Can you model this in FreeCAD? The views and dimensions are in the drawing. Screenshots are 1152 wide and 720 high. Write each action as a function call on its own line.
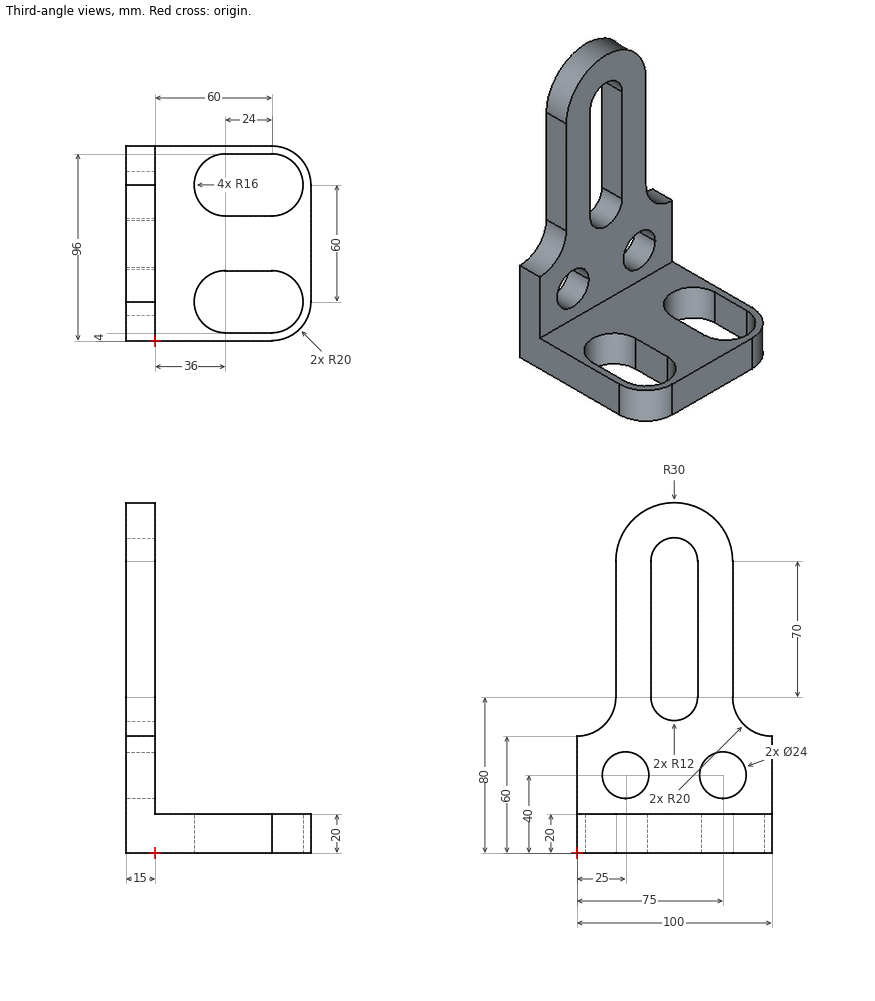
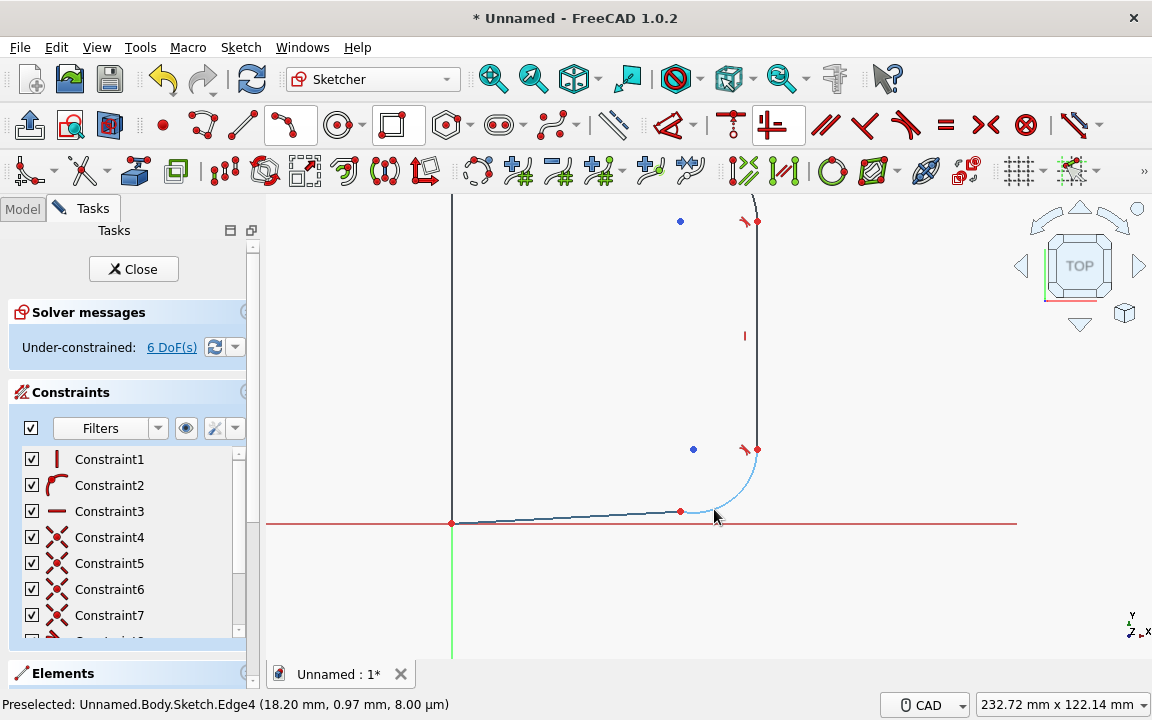
click(714, 509)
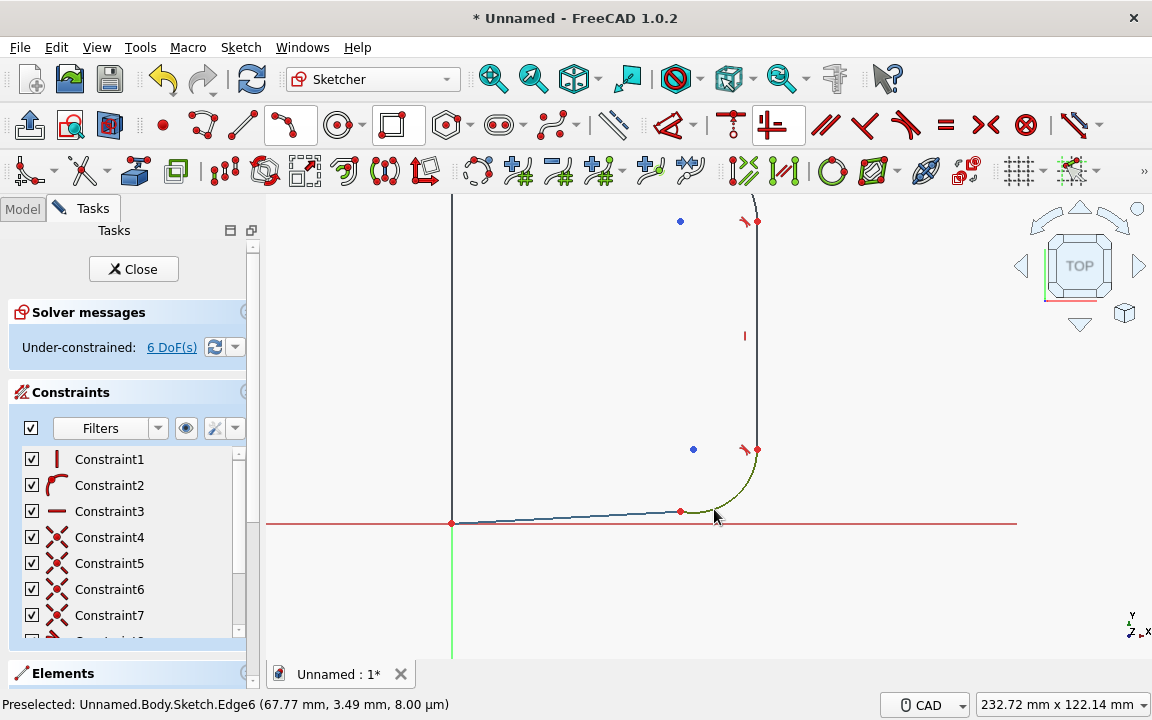
key(t)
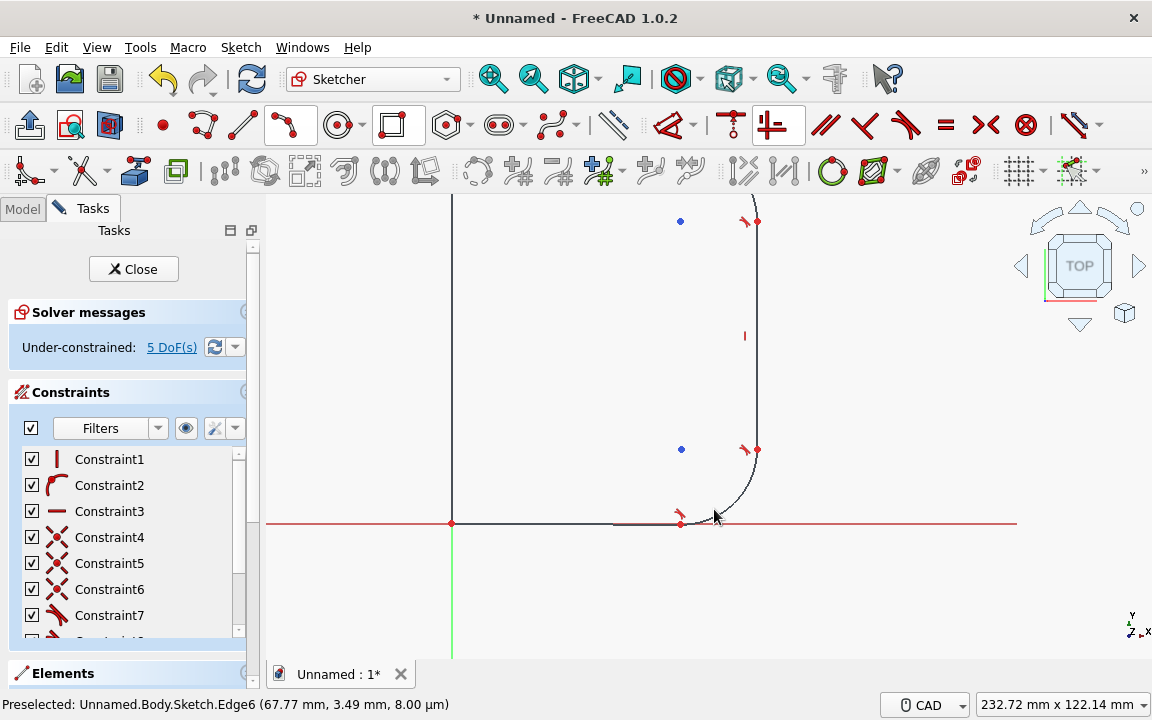
click(521, 524)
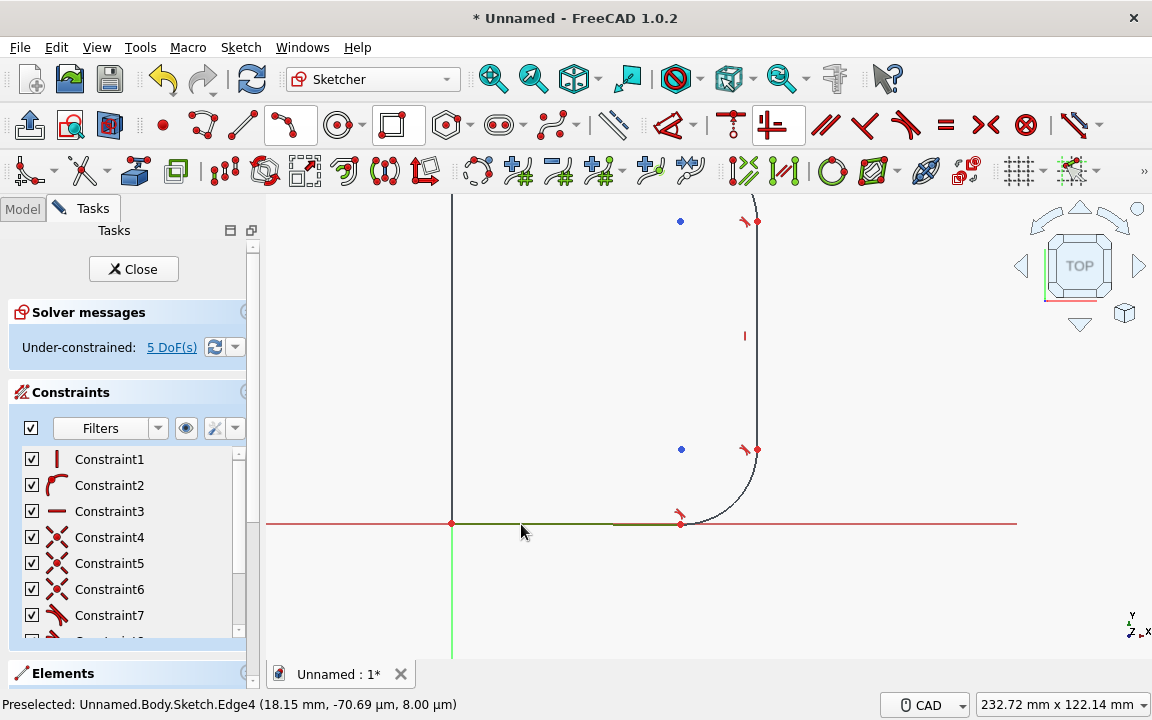
key(h)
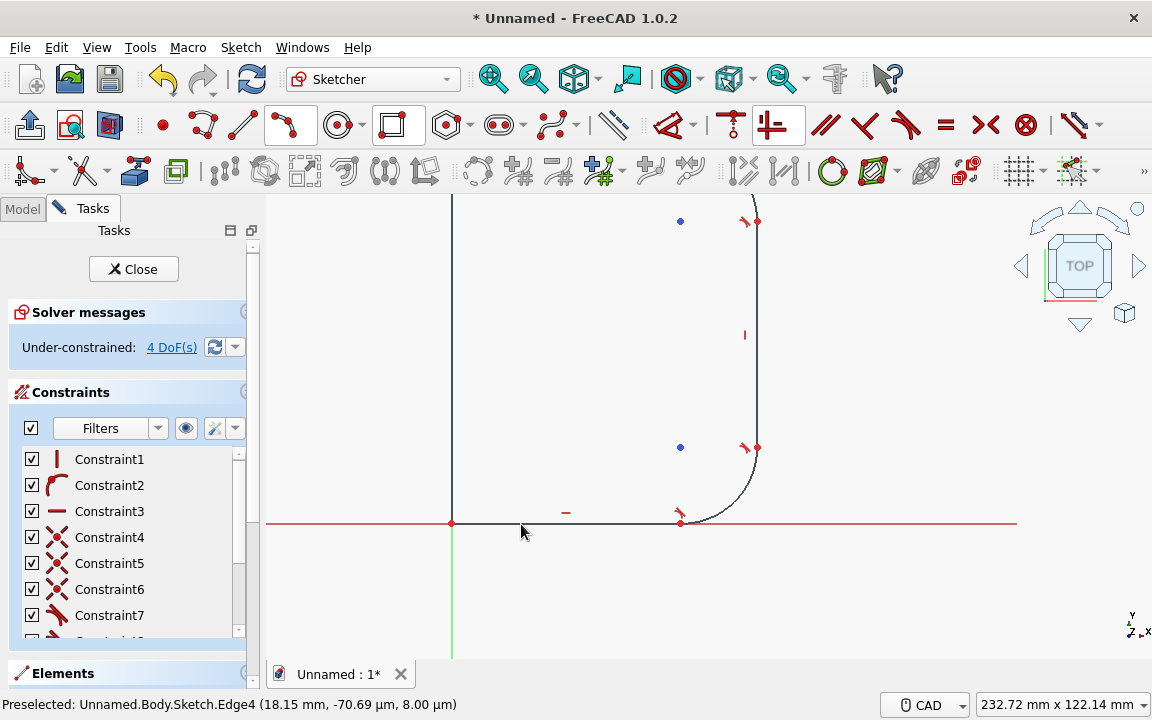
scroll(714, 616, down, 2)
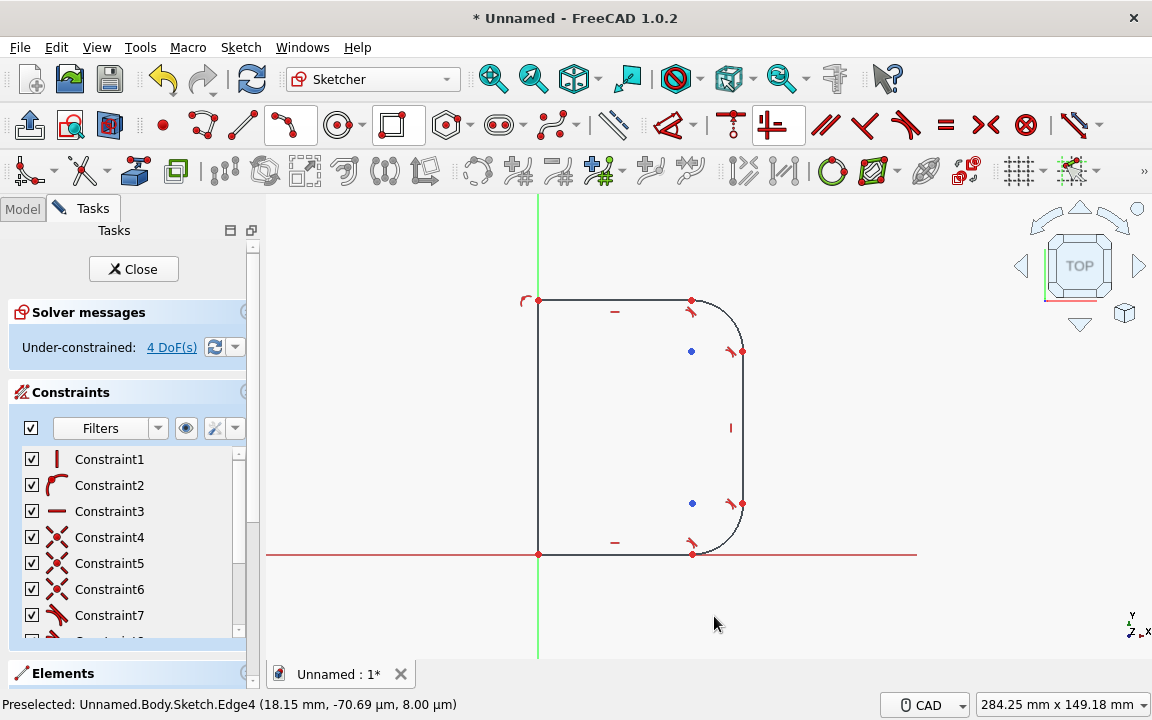
click(737, 328)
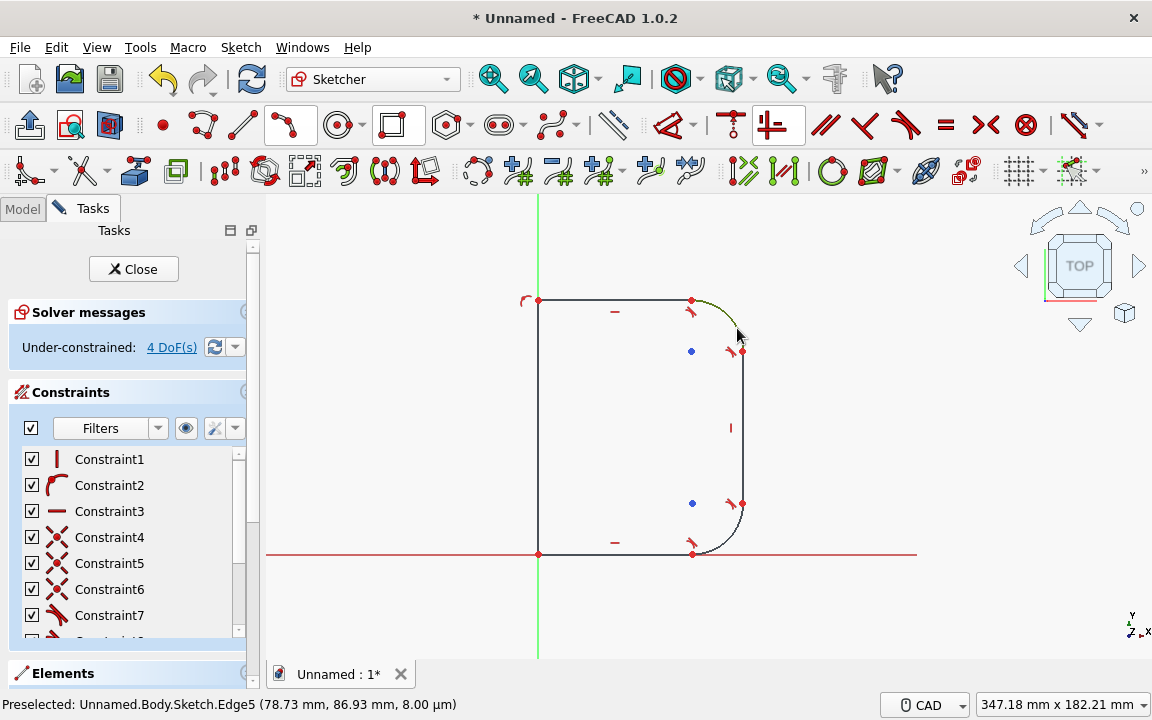
click(737, 527)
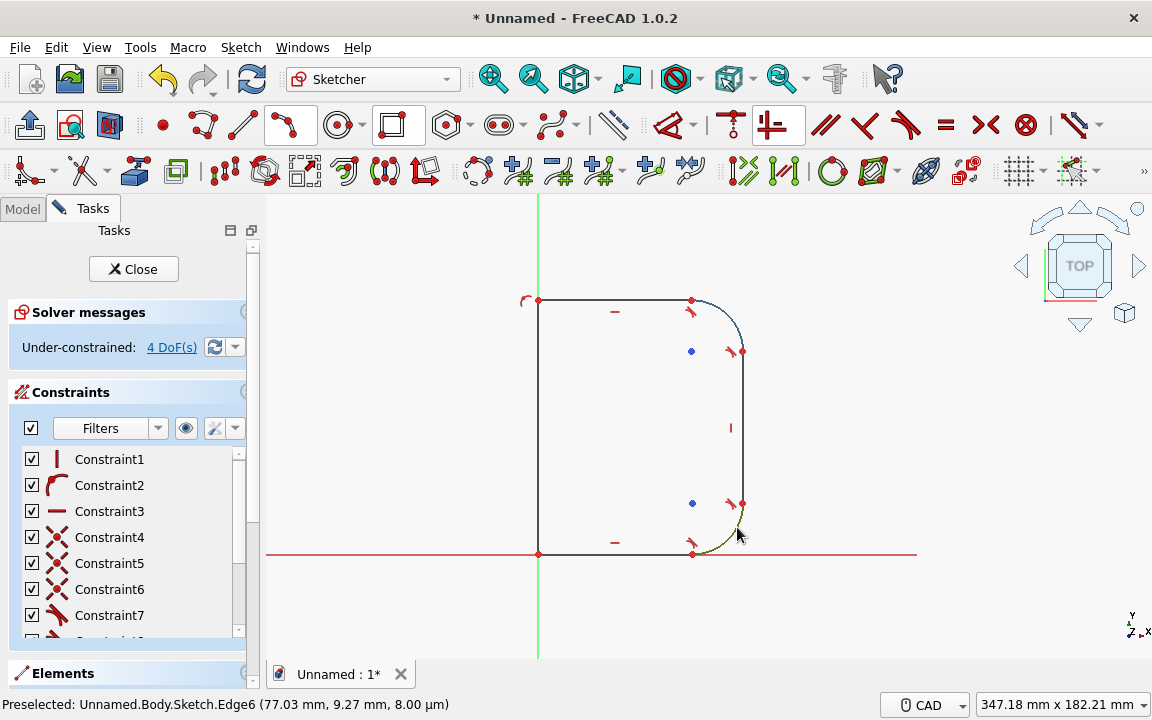
click(946, 126)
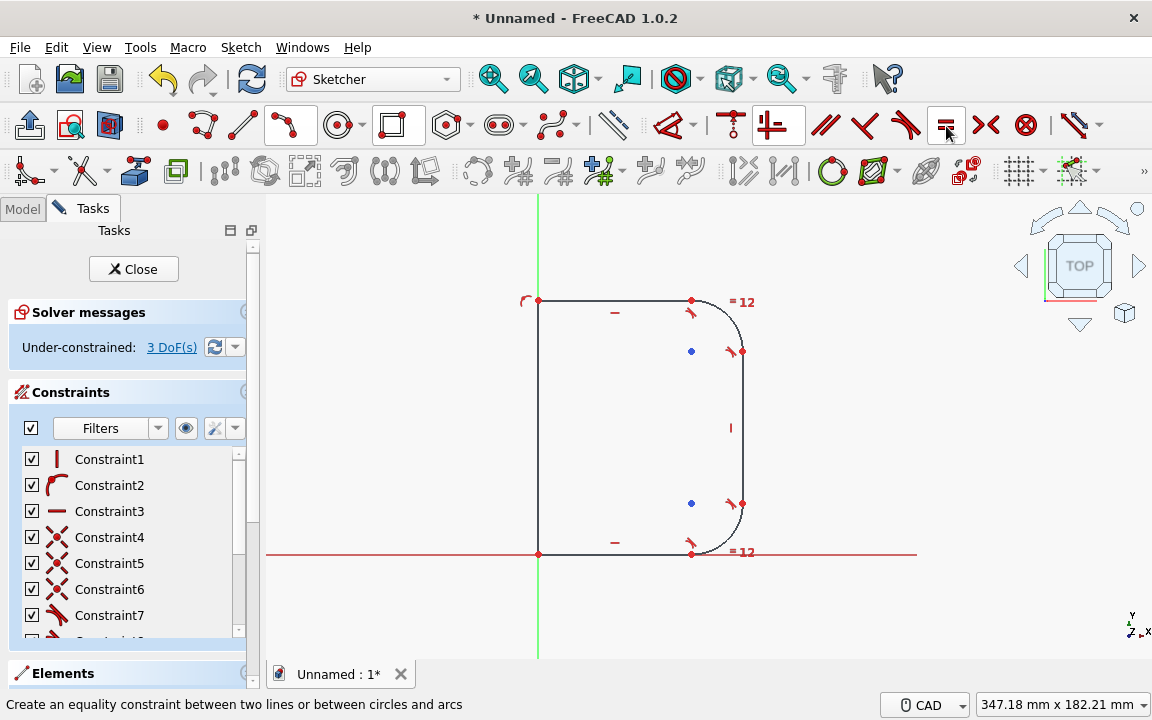
click(668, 126)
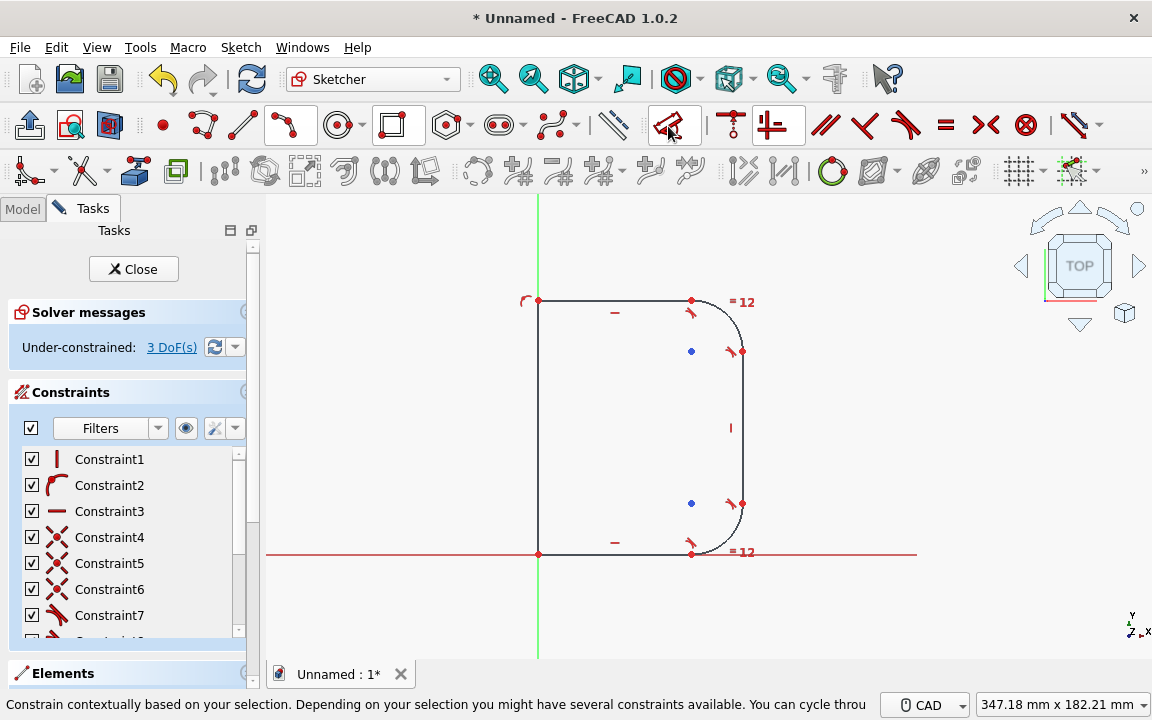
click(737, 328)
click(765, 313)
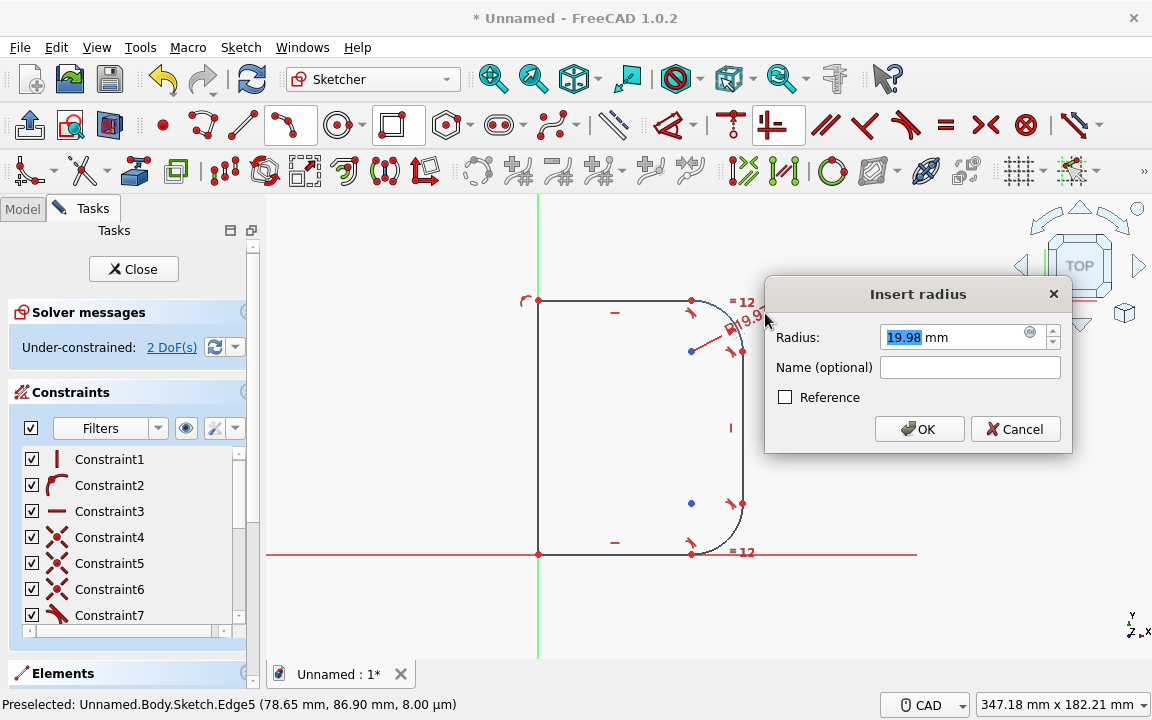
text(20)
key(Return)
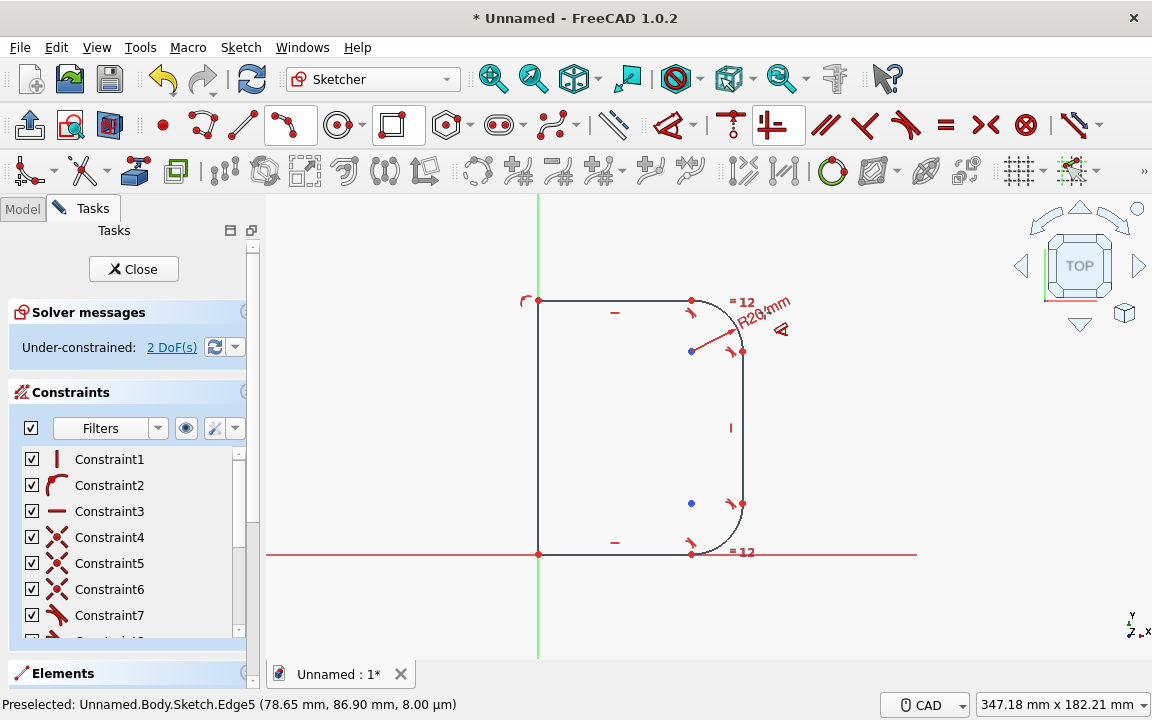
click(743, 458)
click(777, 428)